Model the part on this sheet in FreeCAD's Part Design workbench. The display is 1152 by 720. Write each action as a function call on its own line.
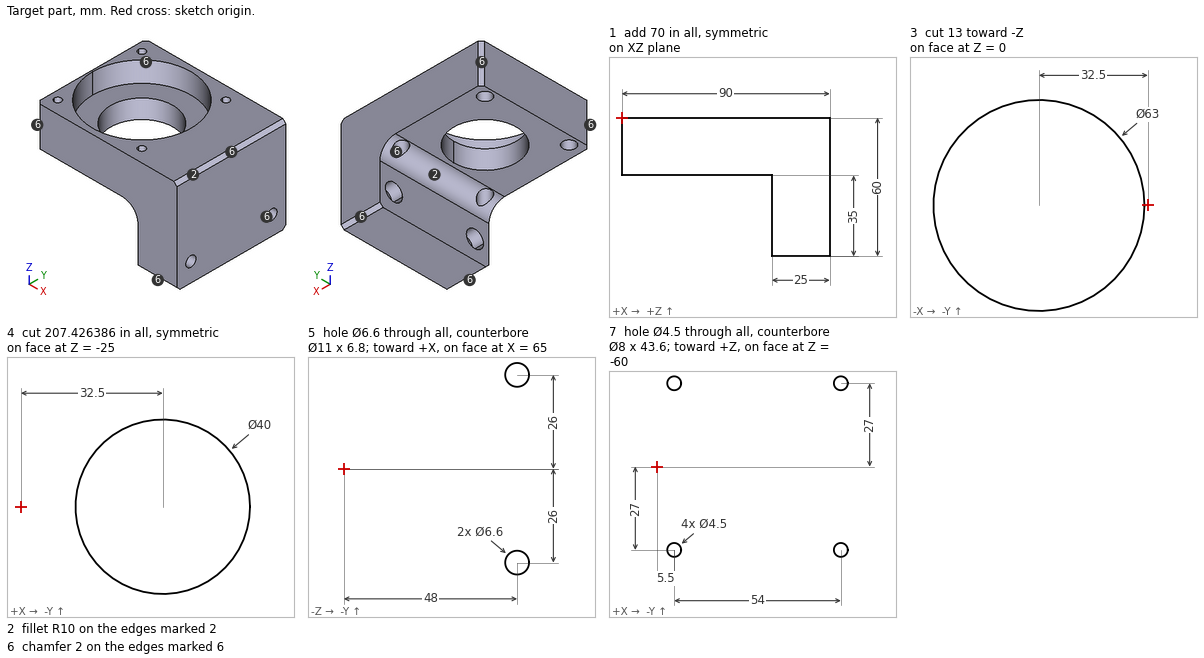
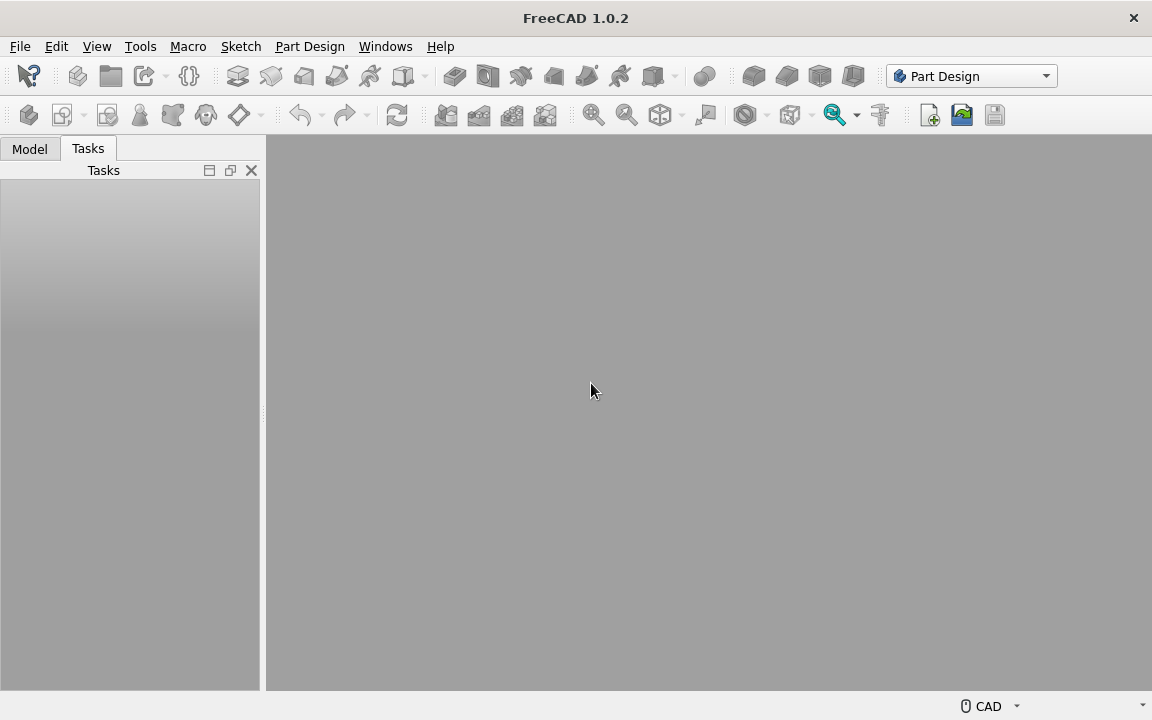
click(929, 116)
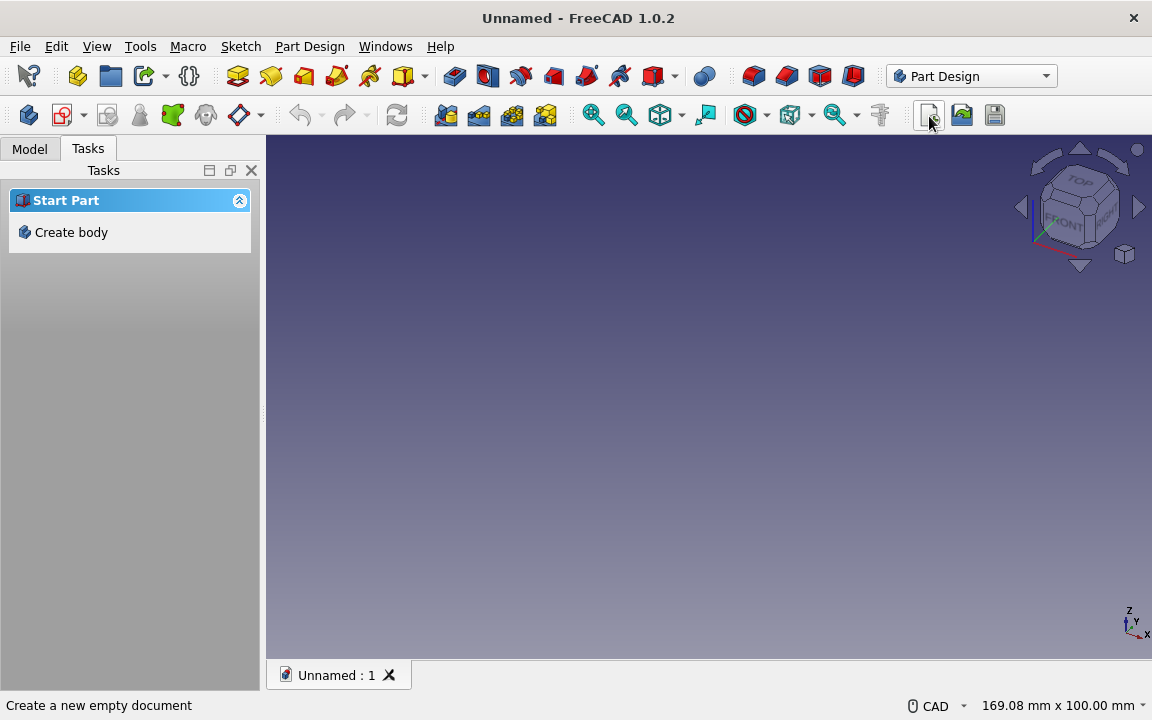
click(62, 116)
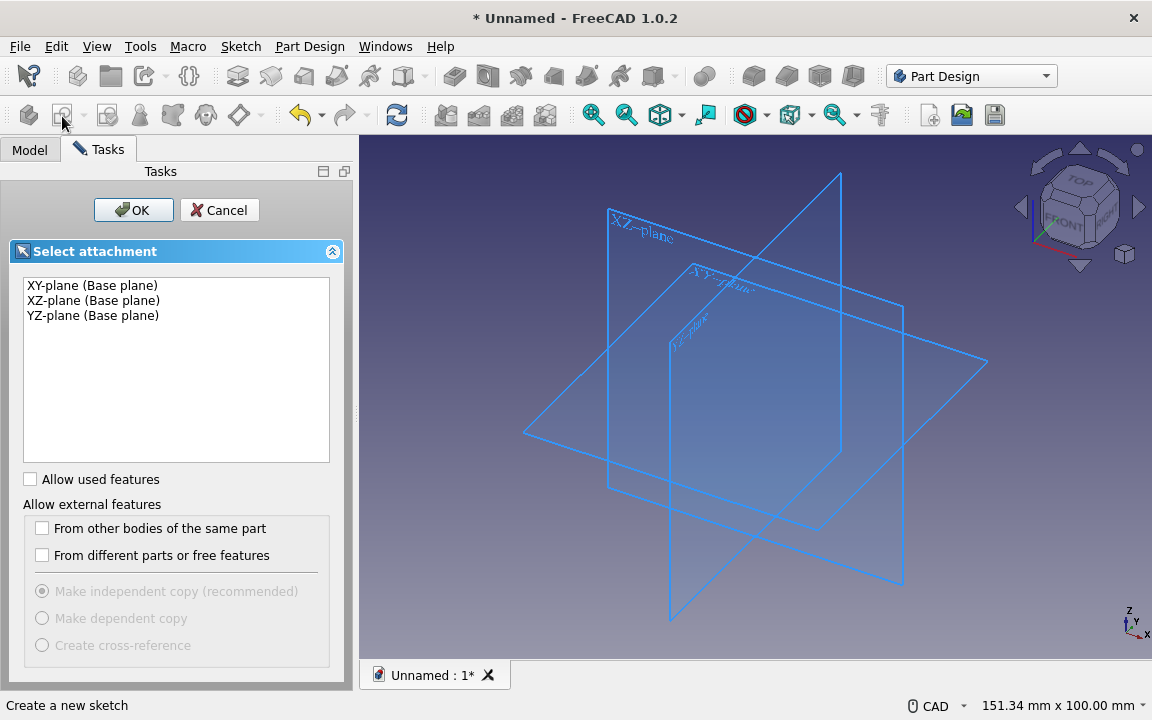
click(84, 300)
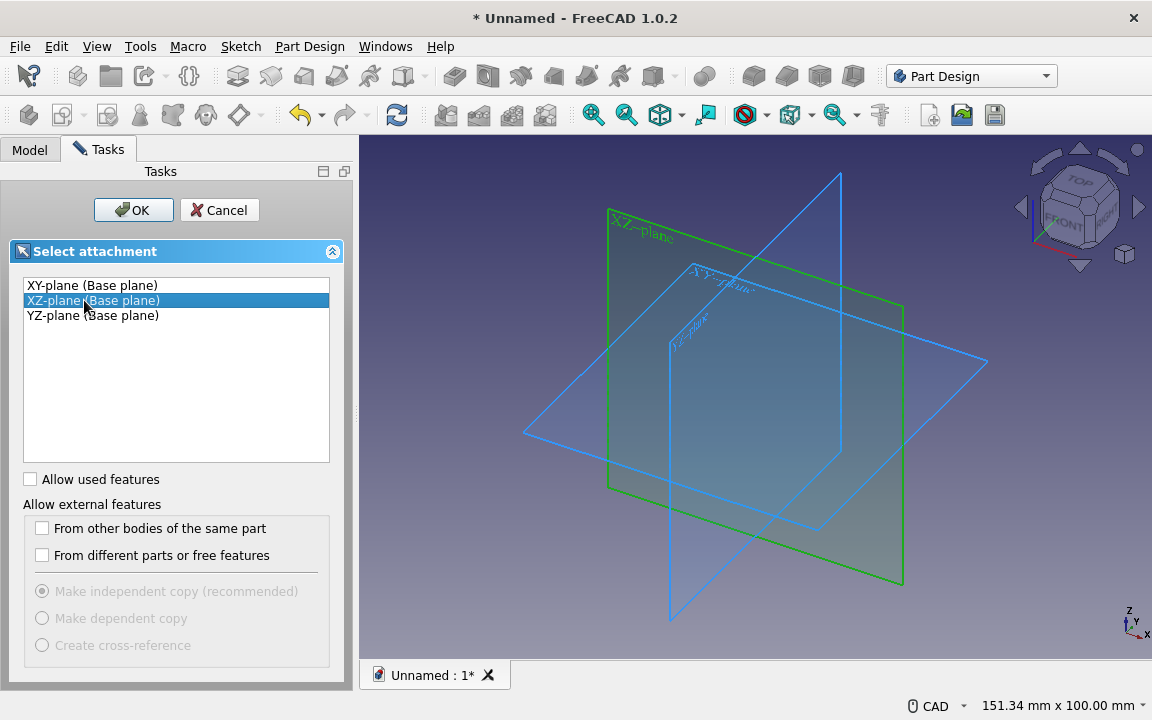
click(134, 210)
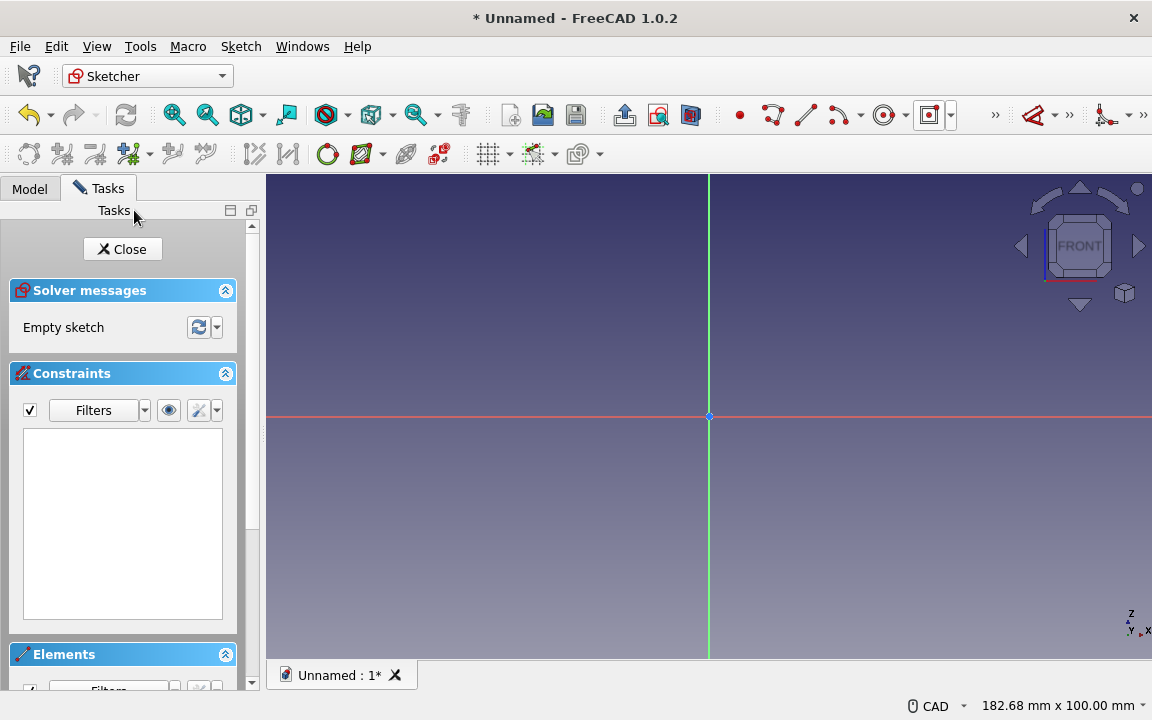
scroll(294, 202, down, 2)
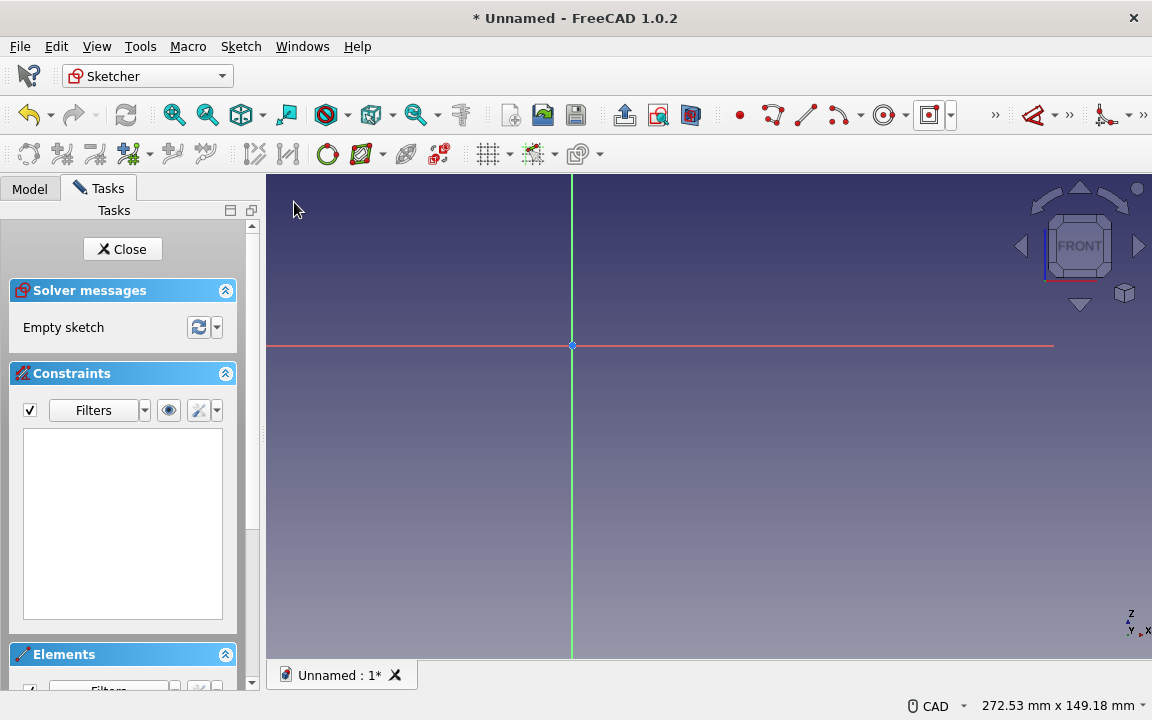
scroll(877, 498, up, 2)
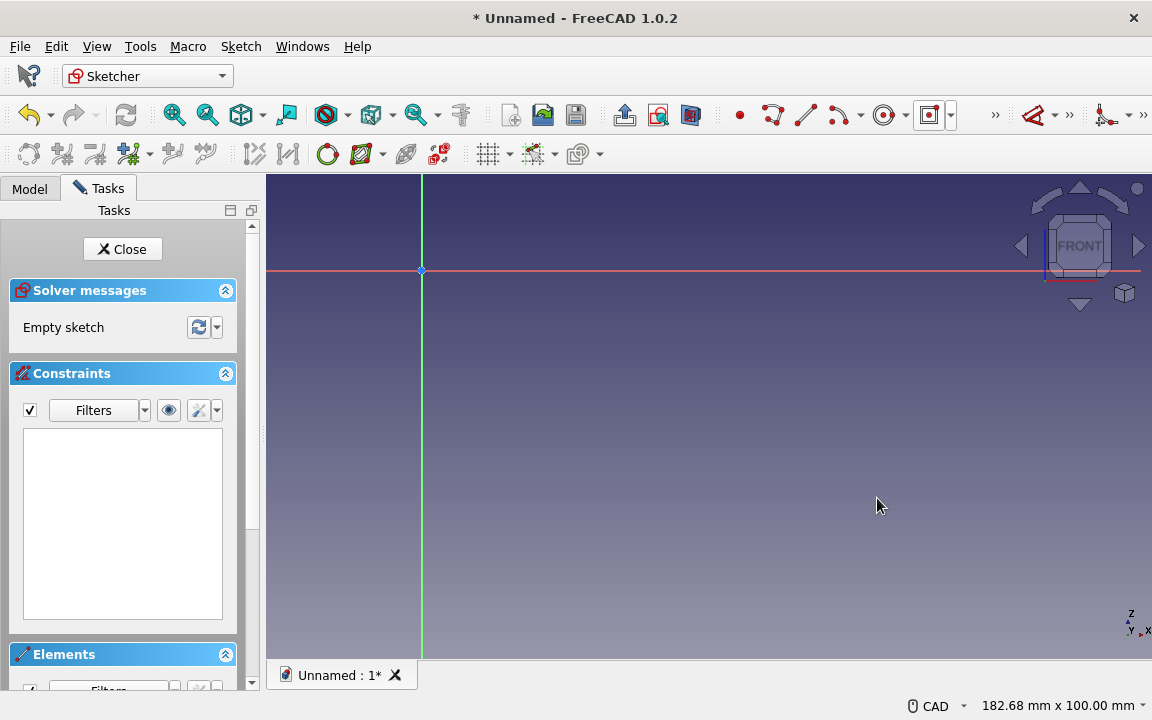
key(g)
key(m)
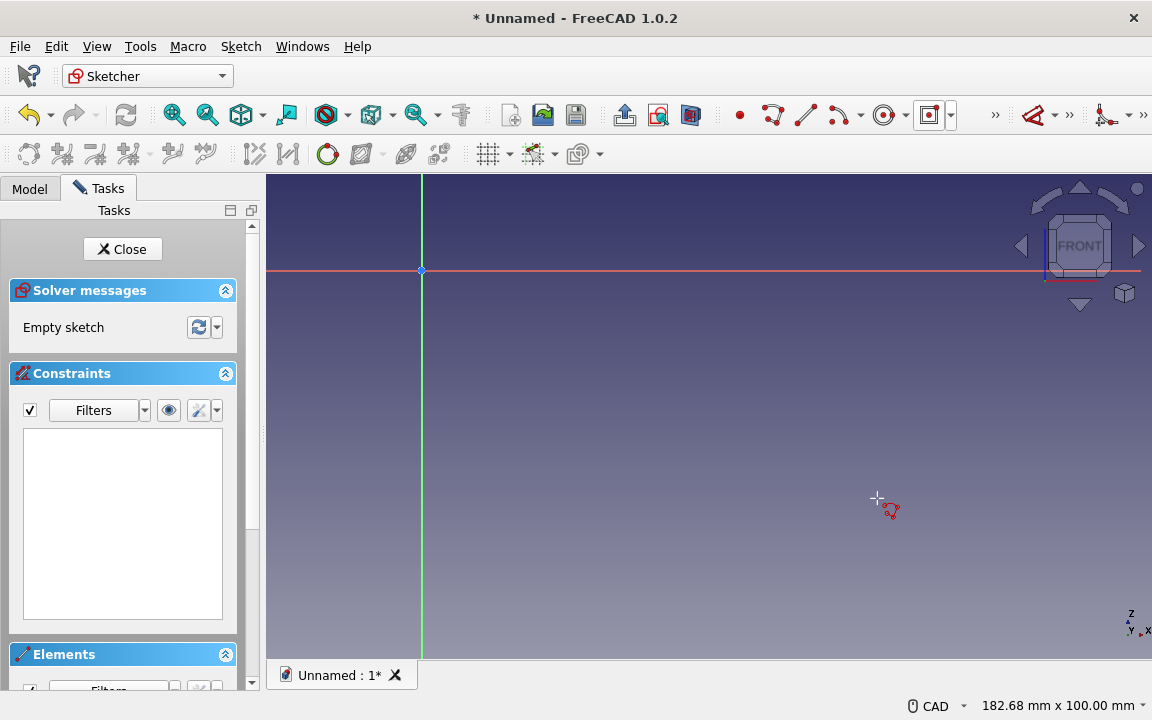
click(422, 271)
click(858, 280)
click(858, 562)
click(737, 562)
click(737, 392)
click(431, 392)
click(422, 271)
key(Escape)
key(Escape)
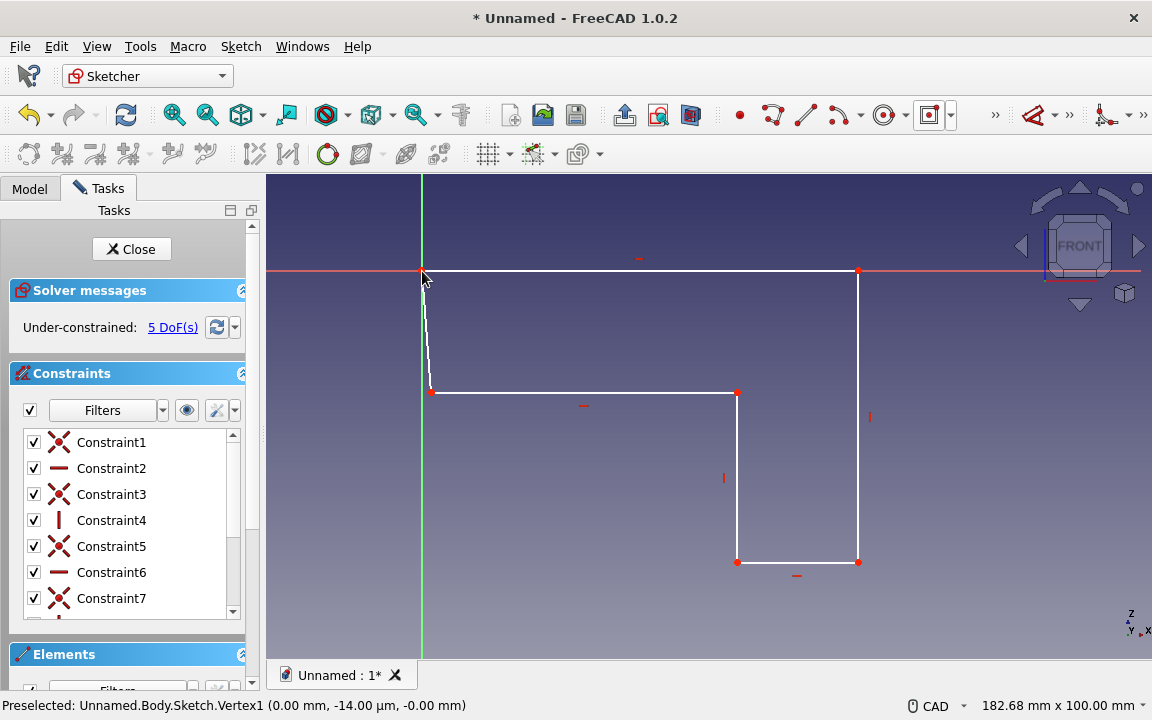
click(425, 307)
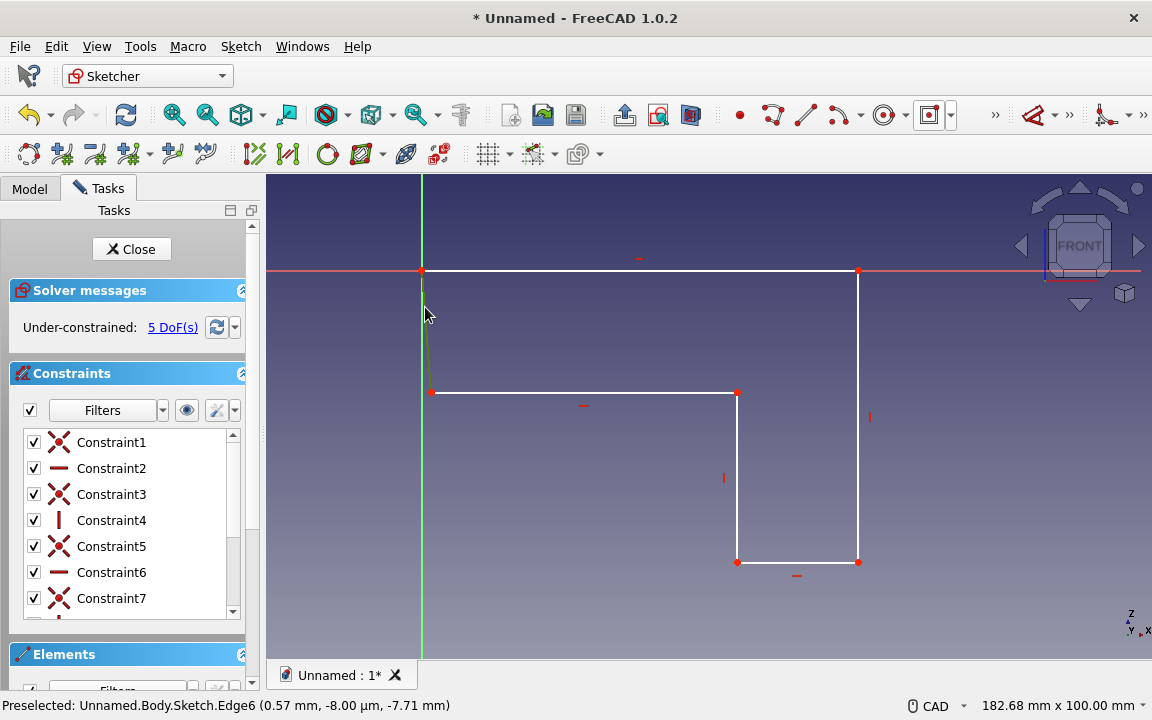
key(v)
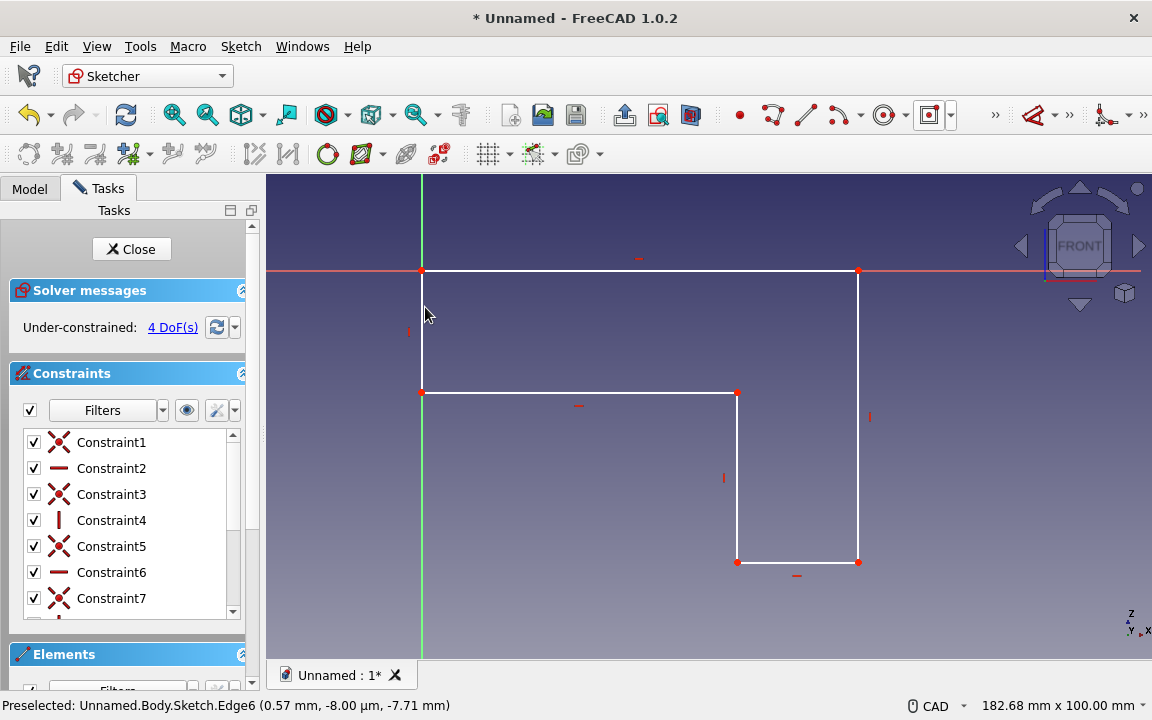
click(1032, 116)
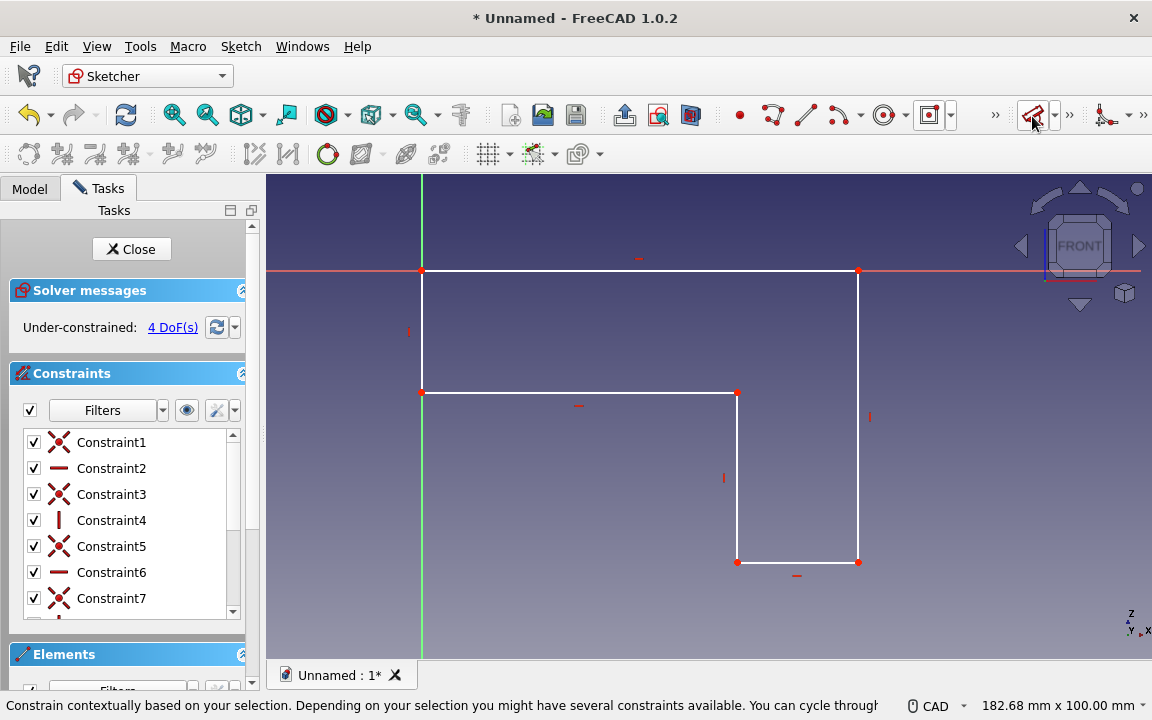
click(553, 271)
click(640, 237)